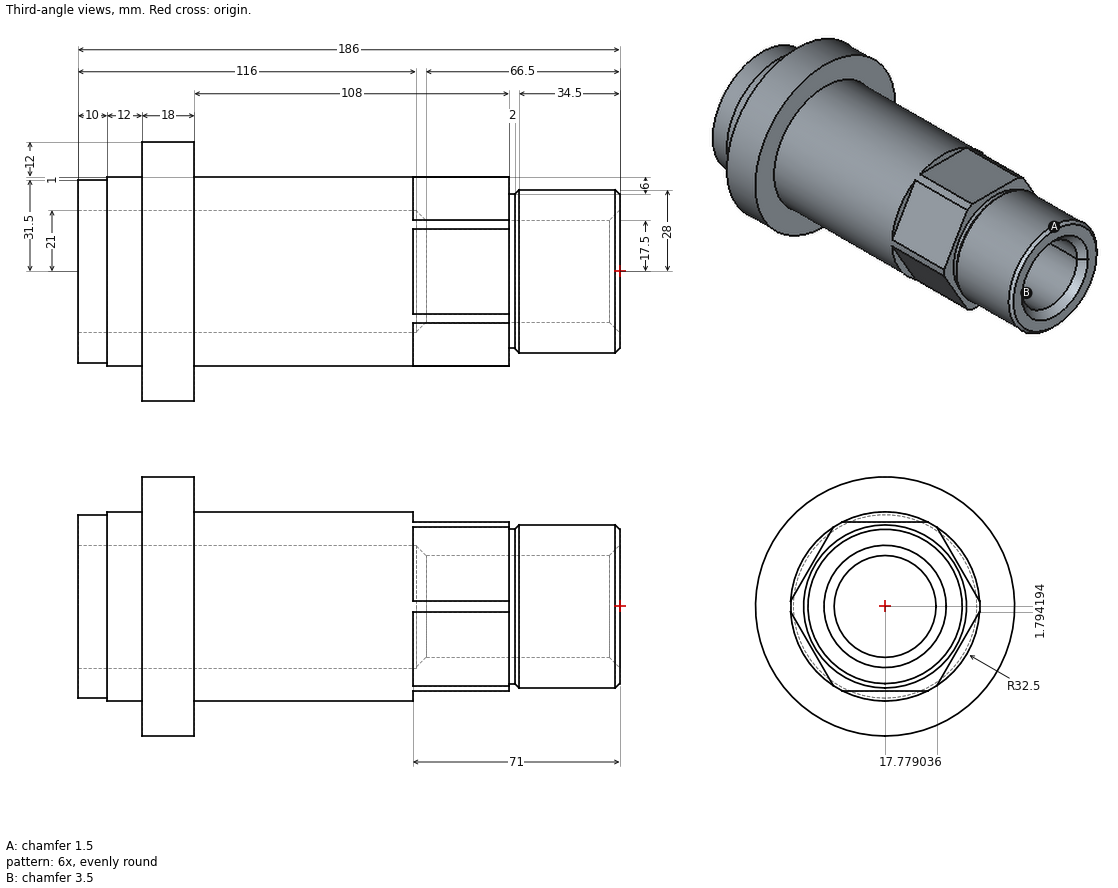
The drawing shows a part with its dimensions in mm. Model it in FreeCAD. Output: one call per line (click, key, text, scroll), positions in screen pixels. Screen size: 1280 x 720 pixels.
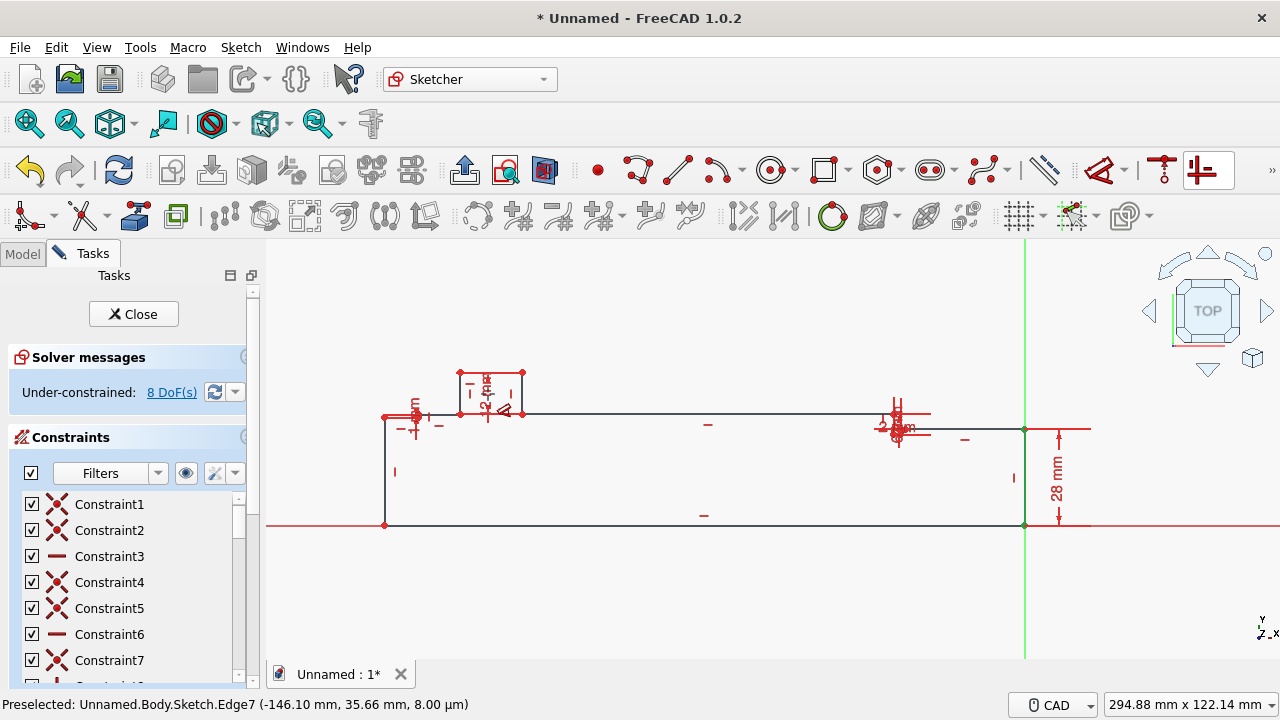
click(504, 373)
click(491, 339)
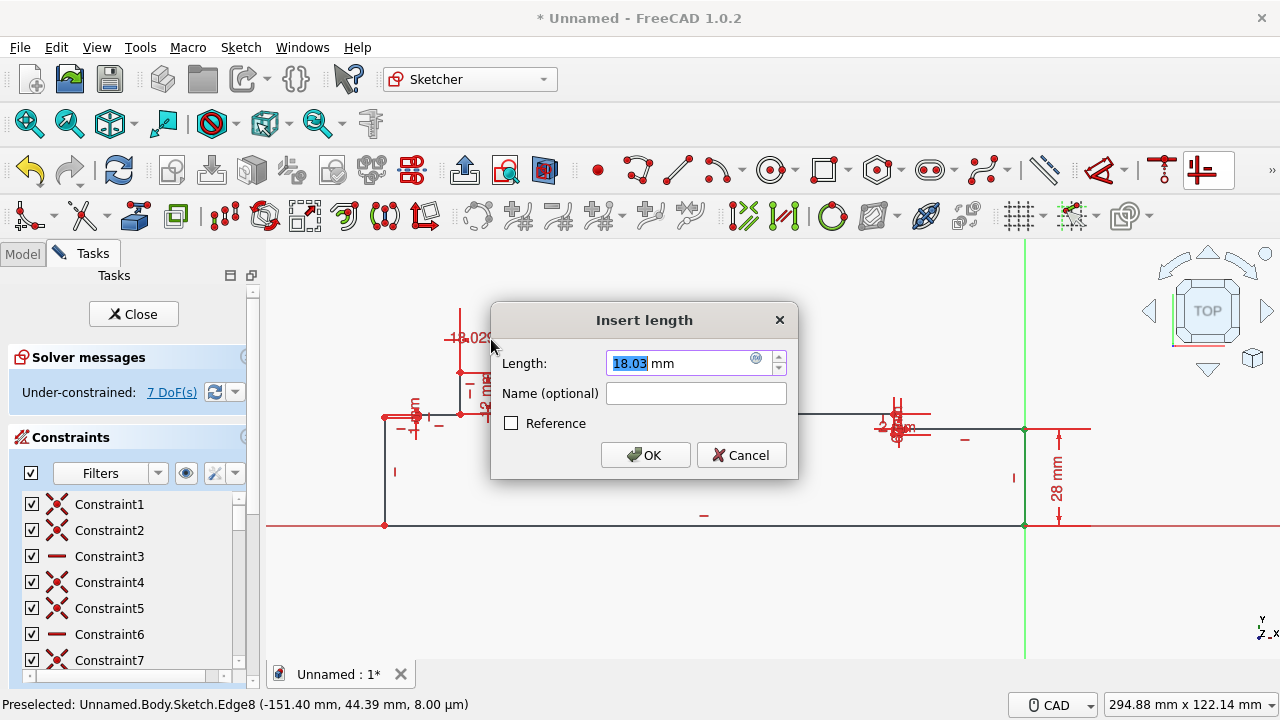
text(18)
key(Return)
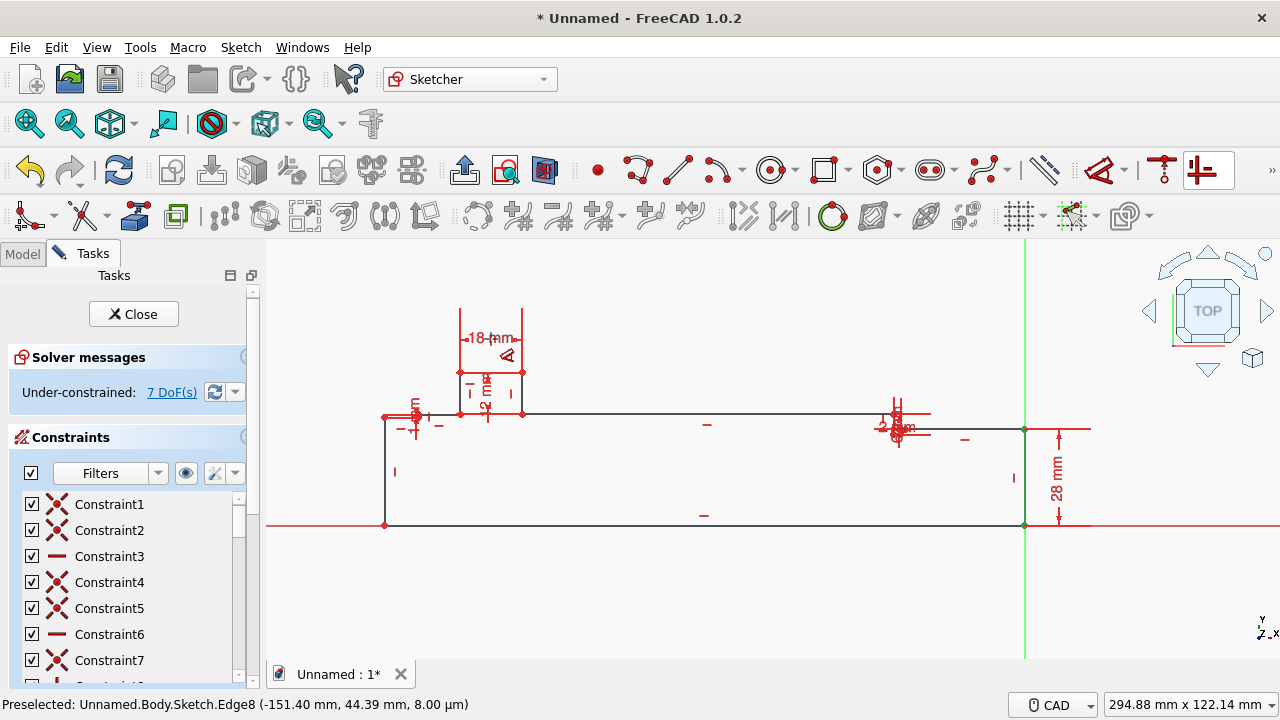
click(460, 385)
click(402, 394)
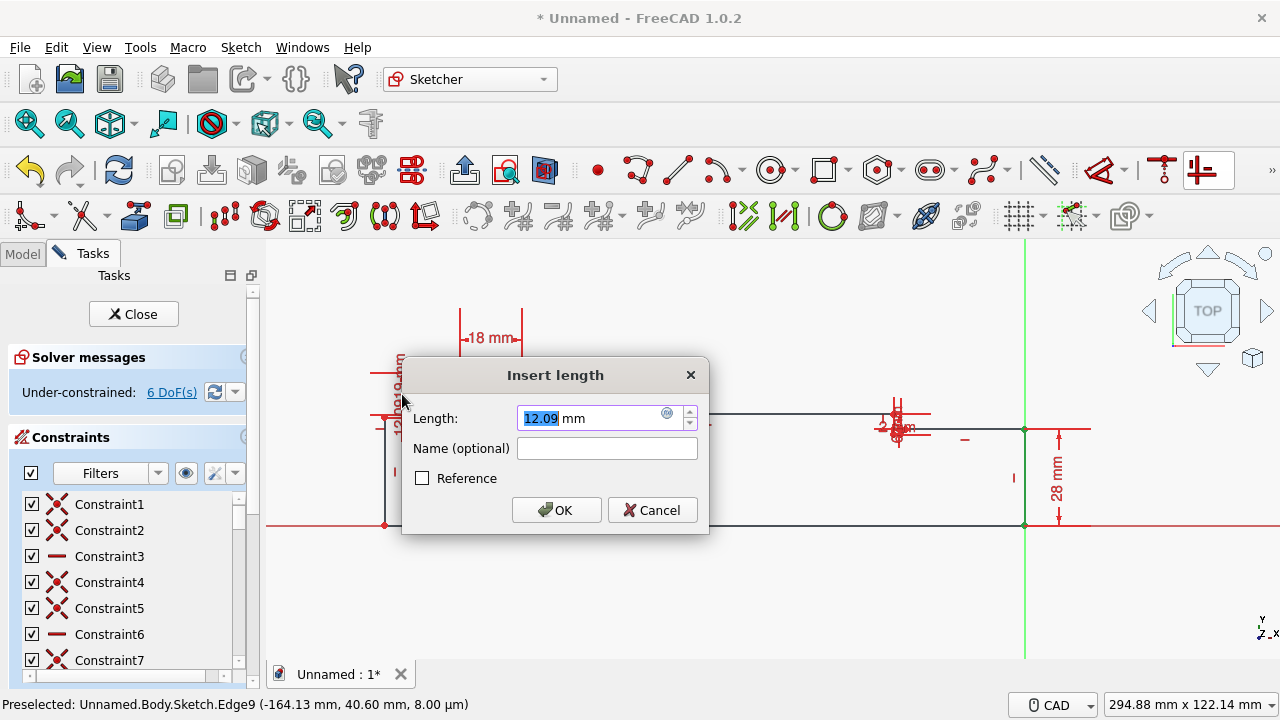
text(12)
key(Return)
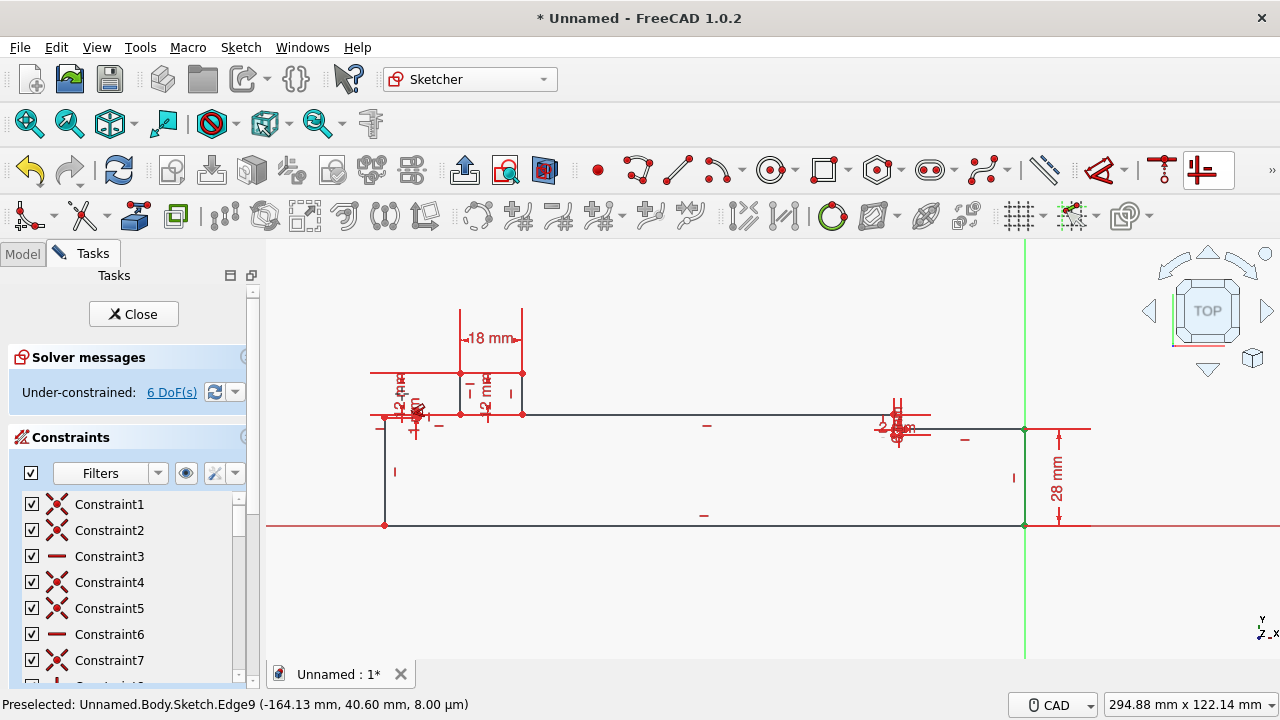
click(448, 415)
click(440, 449)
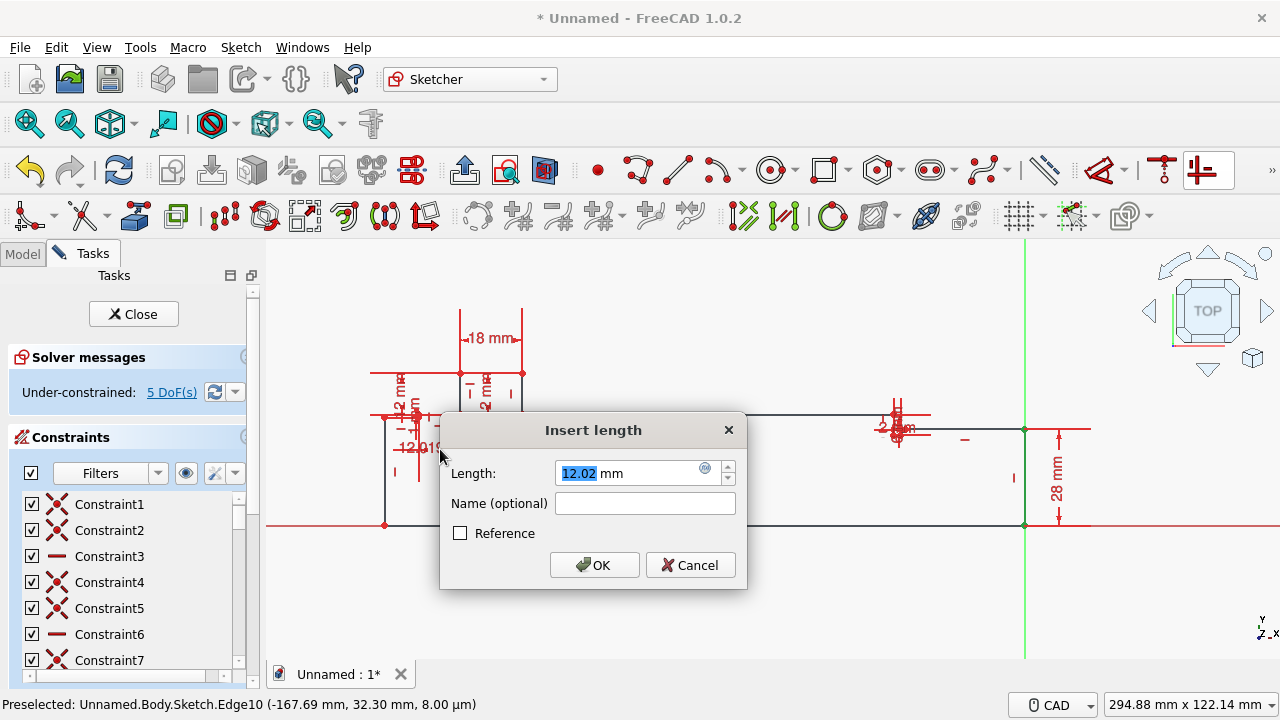
text(12)
key(Return)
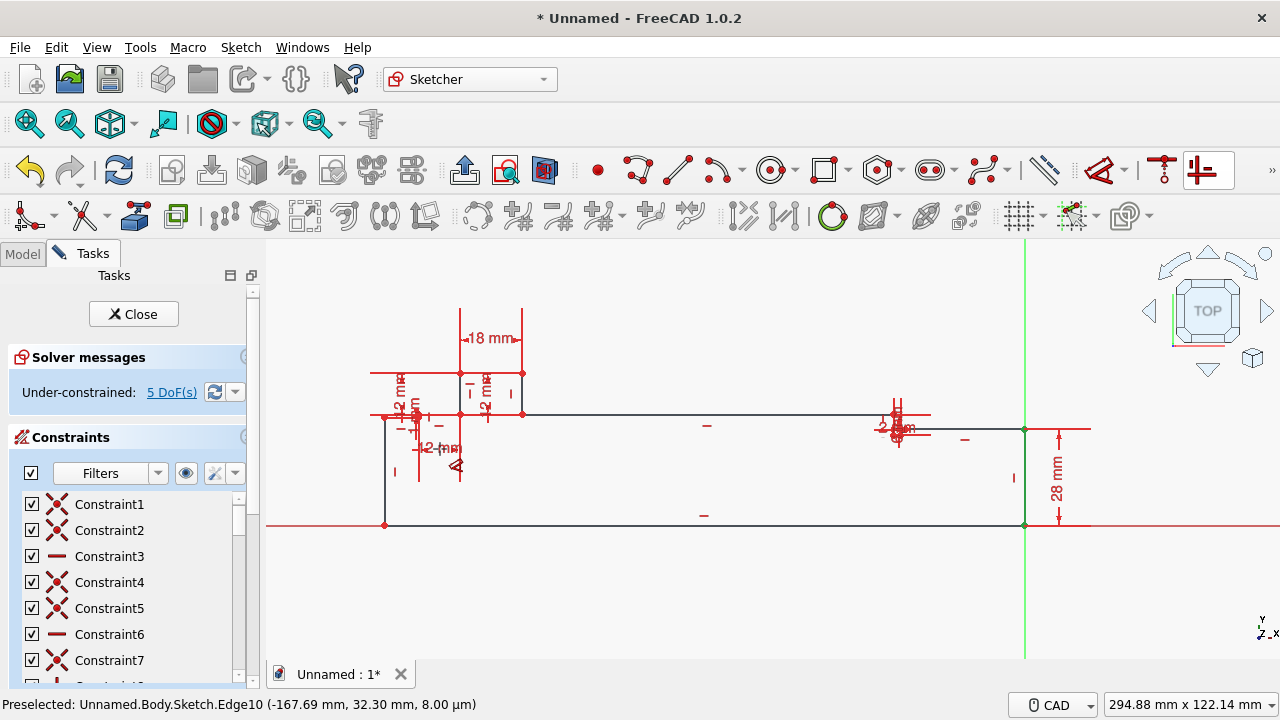
scroll(409, 418, up, 2)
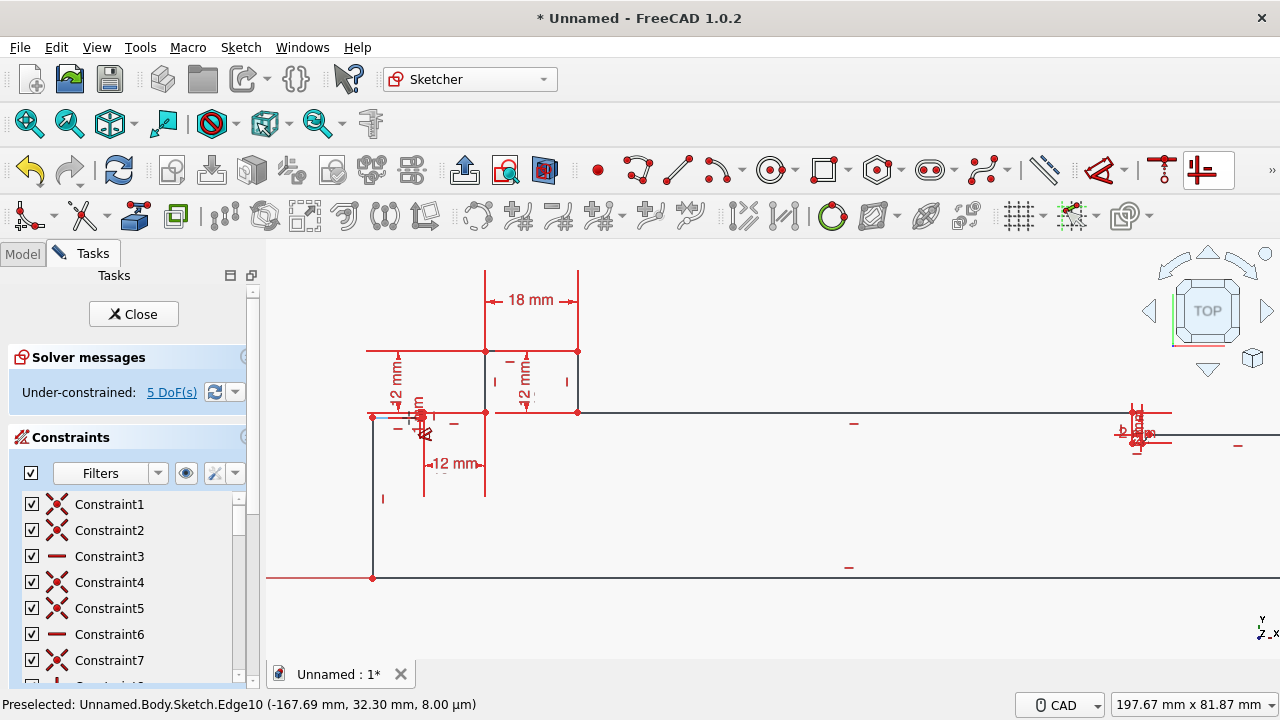
click(408, 418)
click(398, 360)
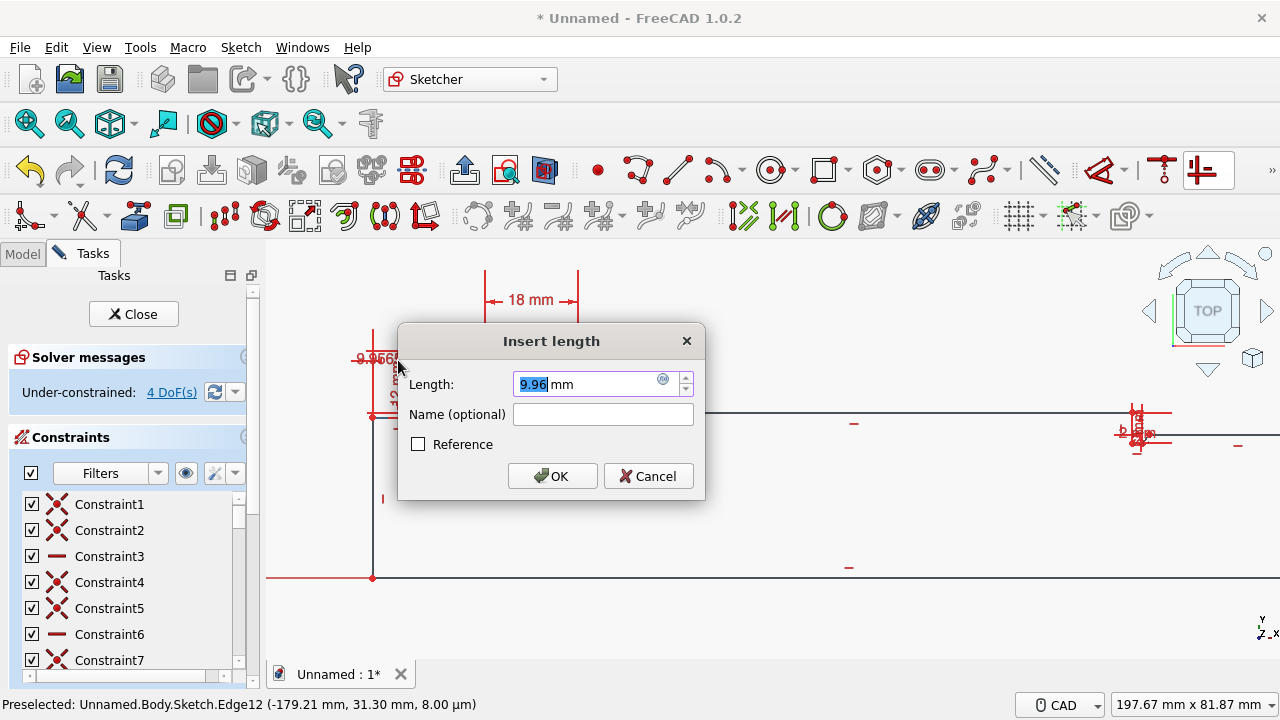
text(10)
key(Return)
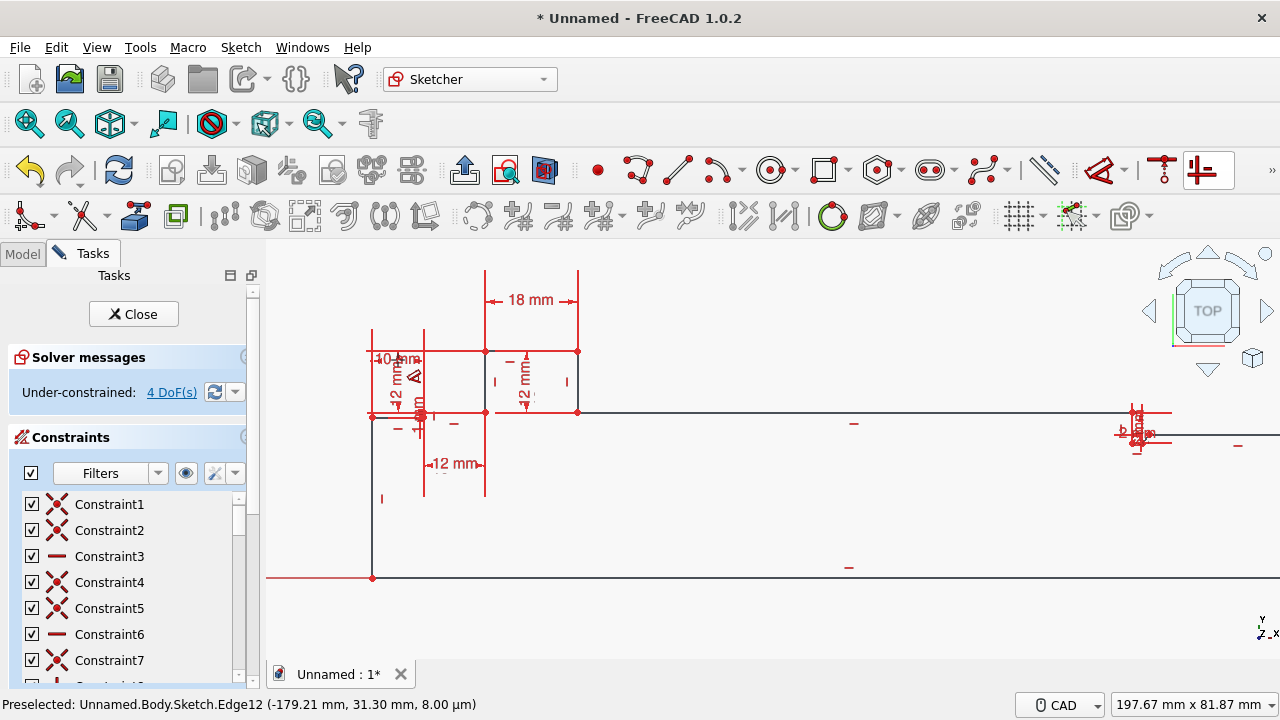
click(966, 413)
click(846, 379)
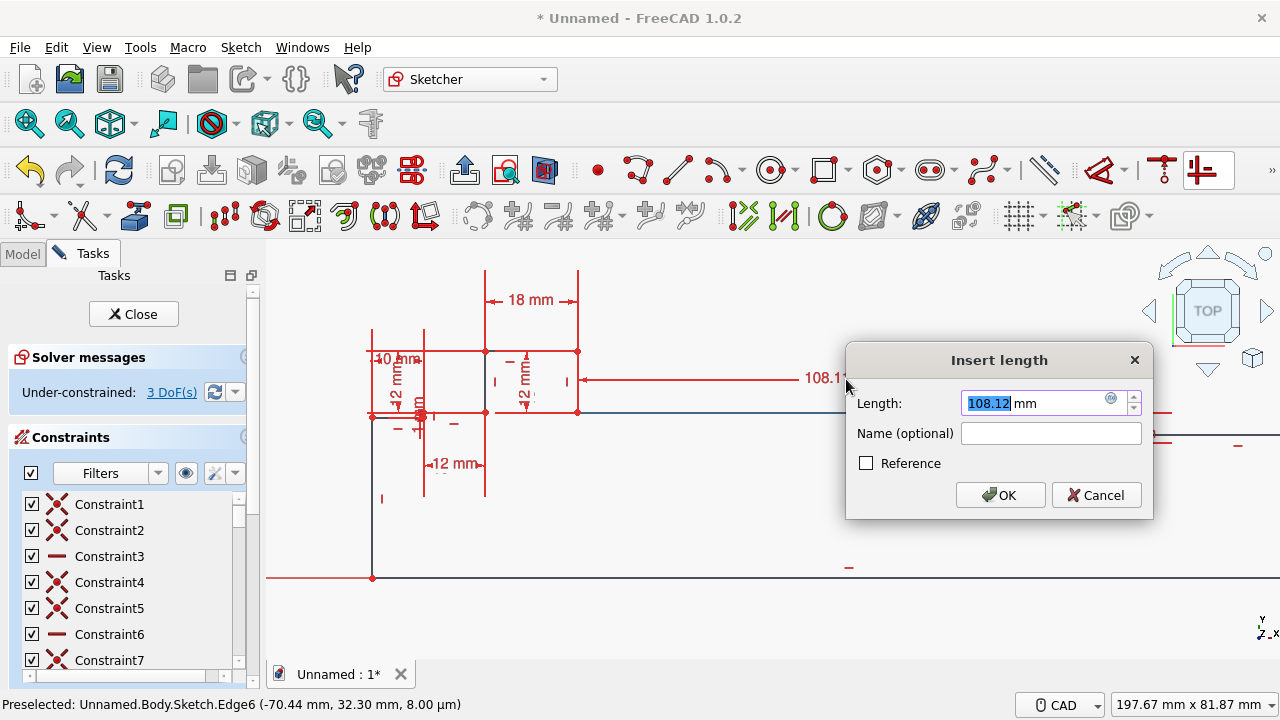
text(108)
key(Return)